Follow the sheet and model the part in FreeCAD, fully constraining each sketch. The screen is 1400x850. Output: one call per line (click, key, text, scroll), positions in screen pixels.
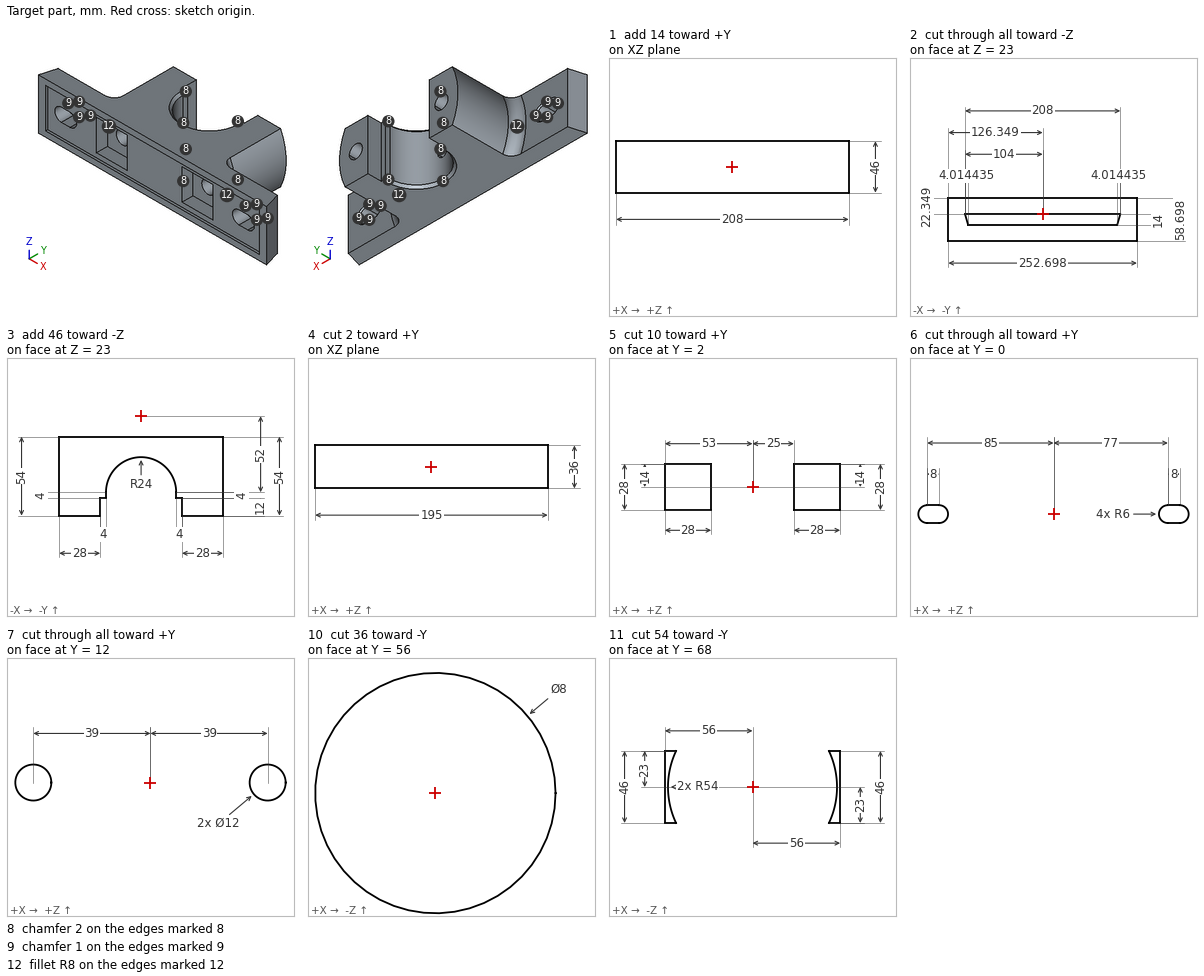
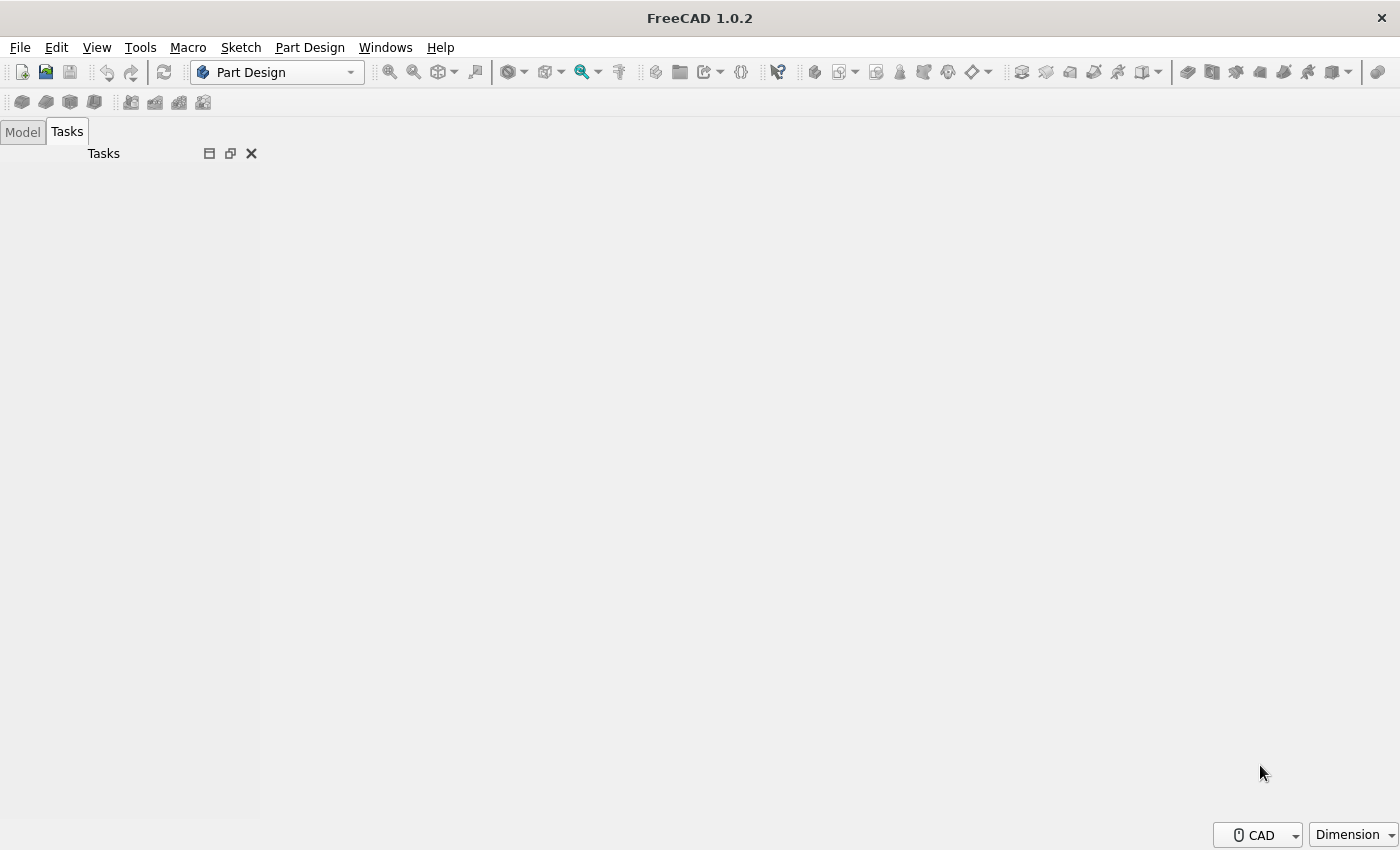
click(22, 72)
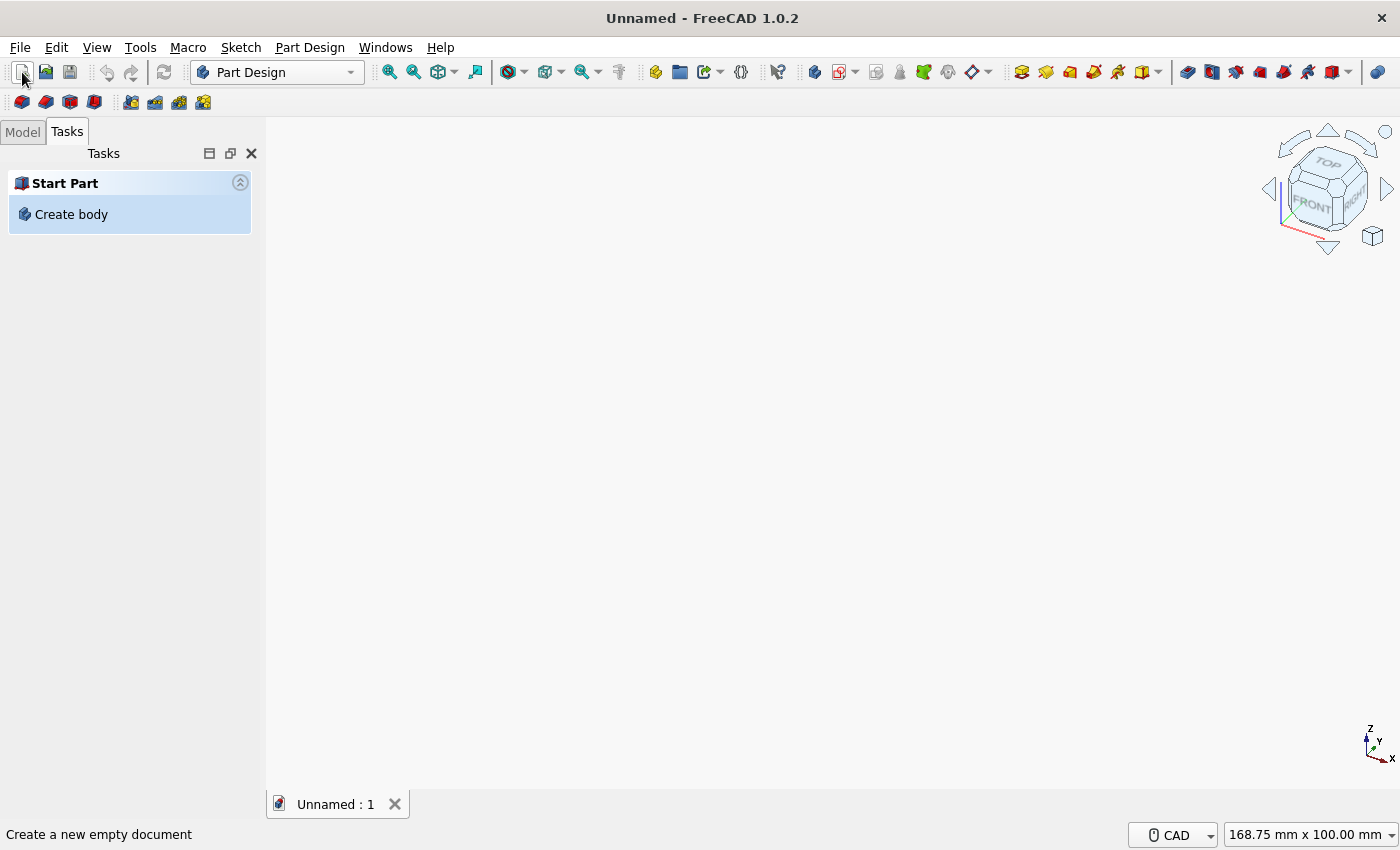
click(840, 72)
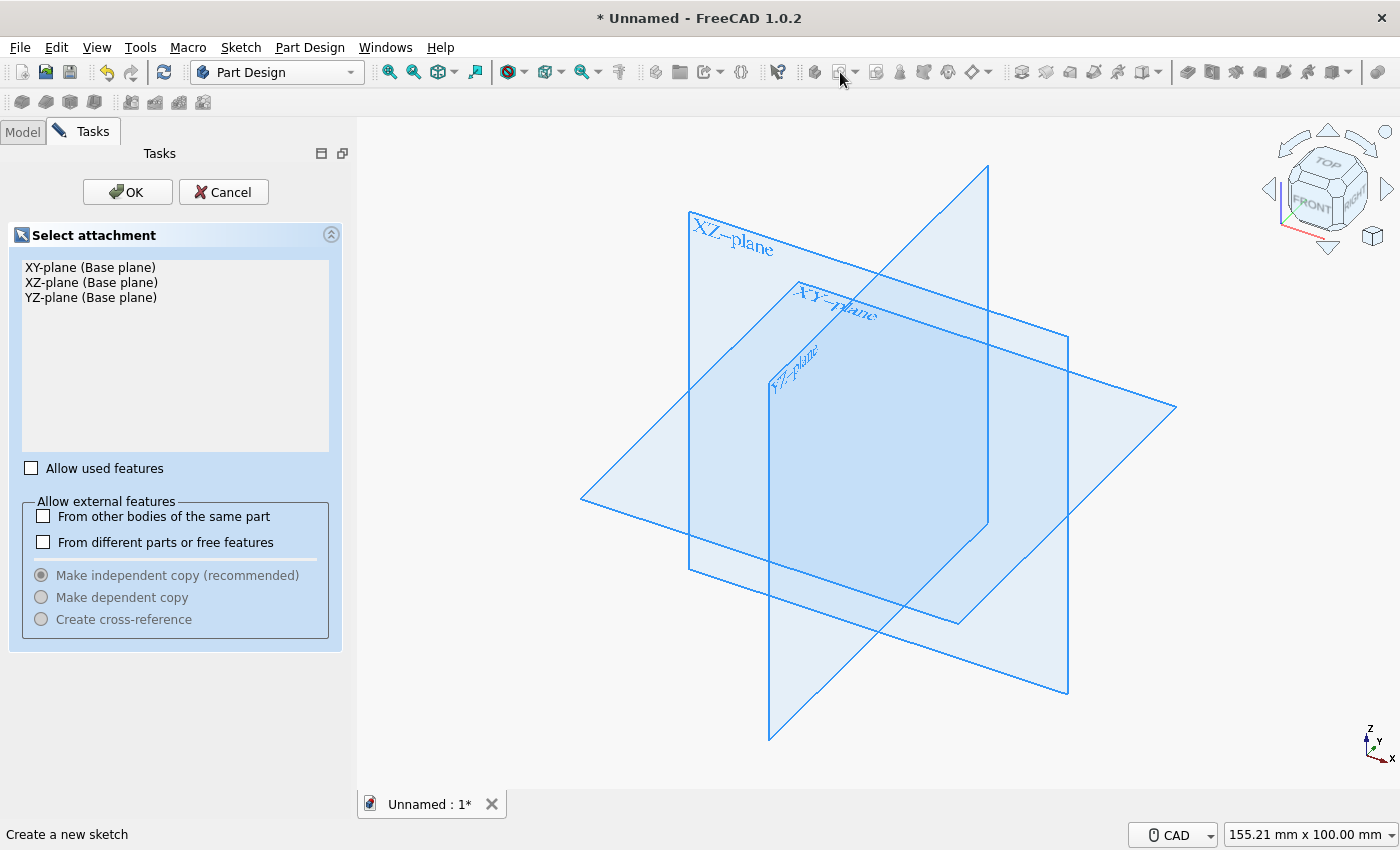
click(82, 282)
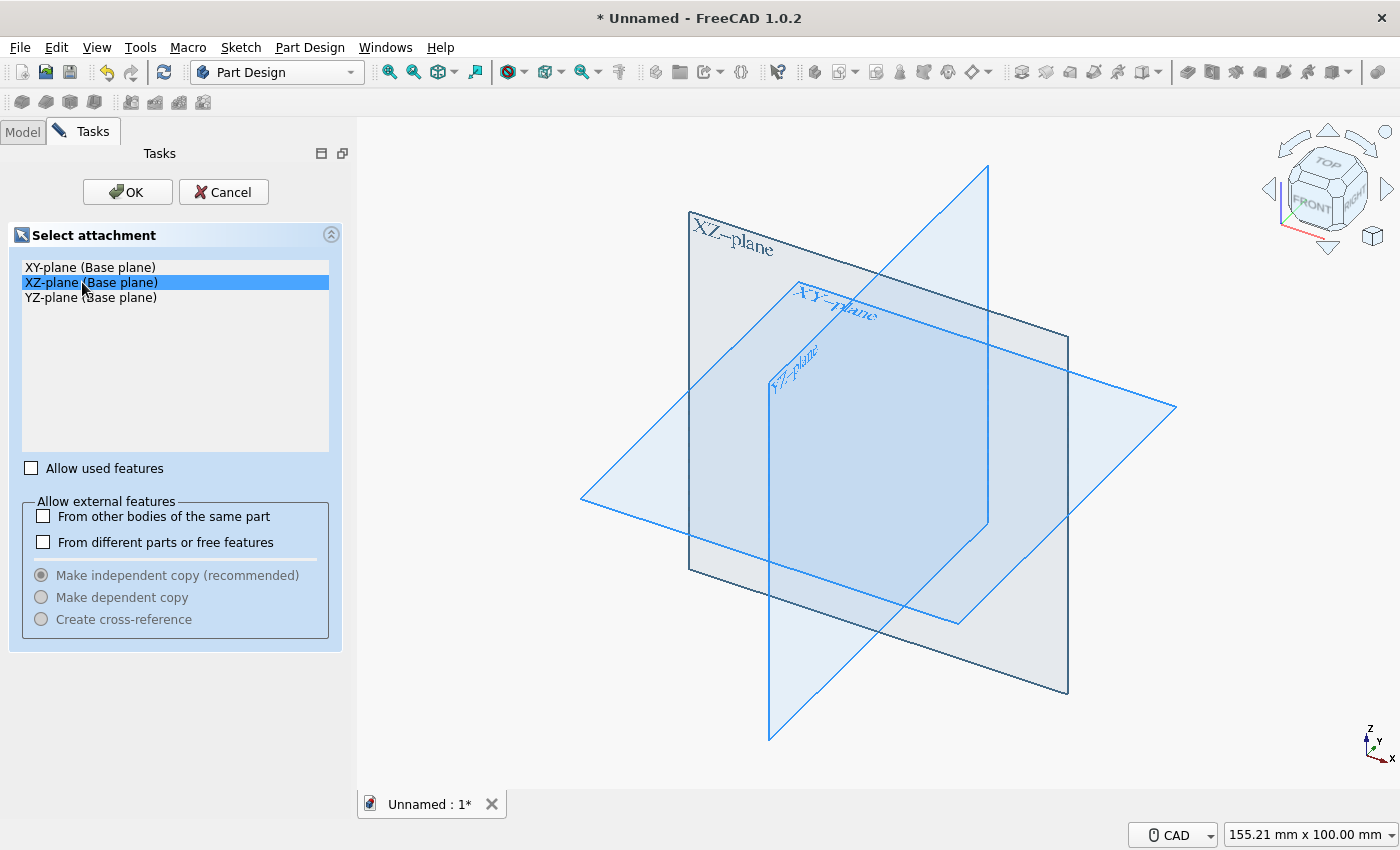
click(128, 192)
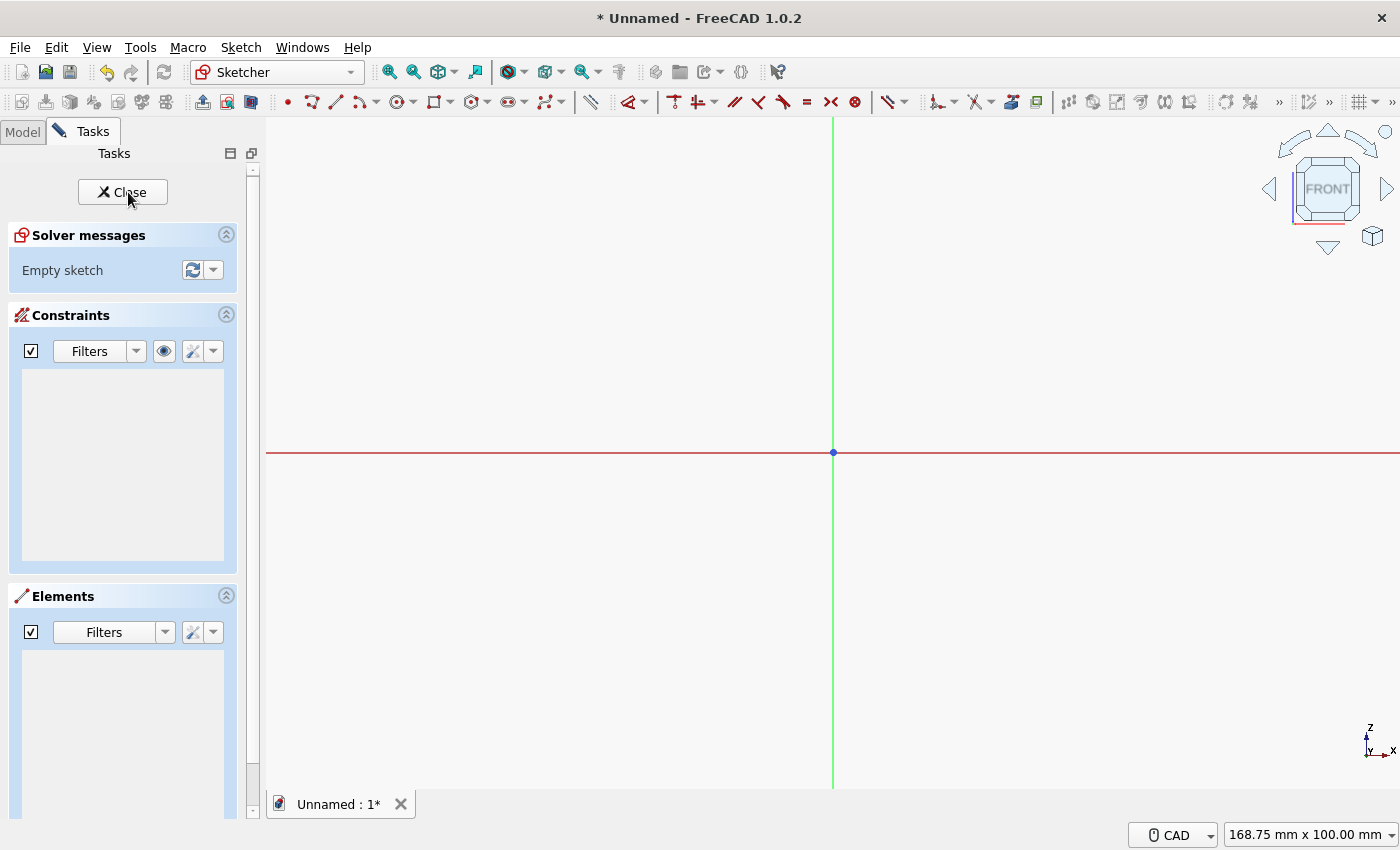
scroll(709, 453, down, 4)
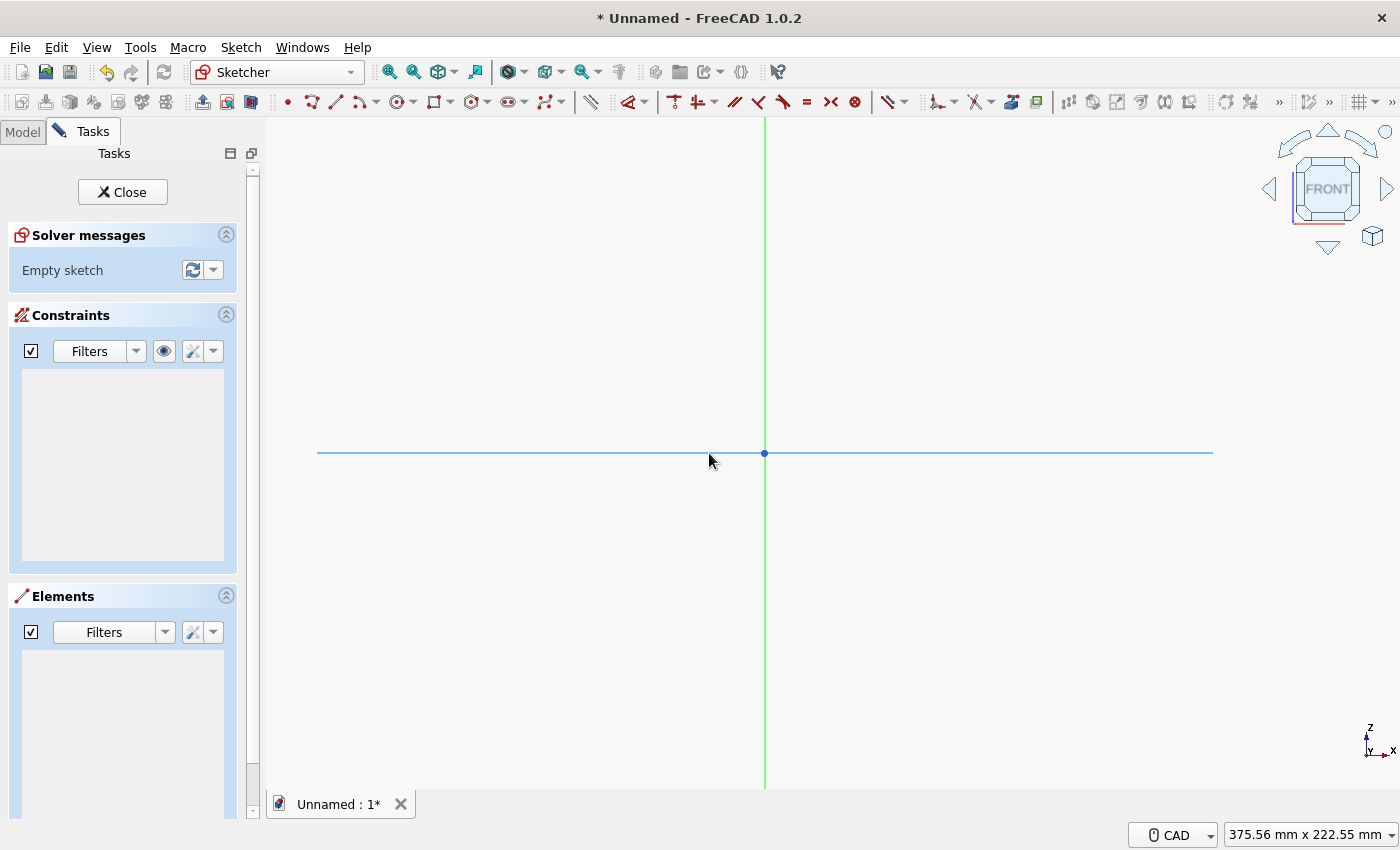
key(g)
key(v)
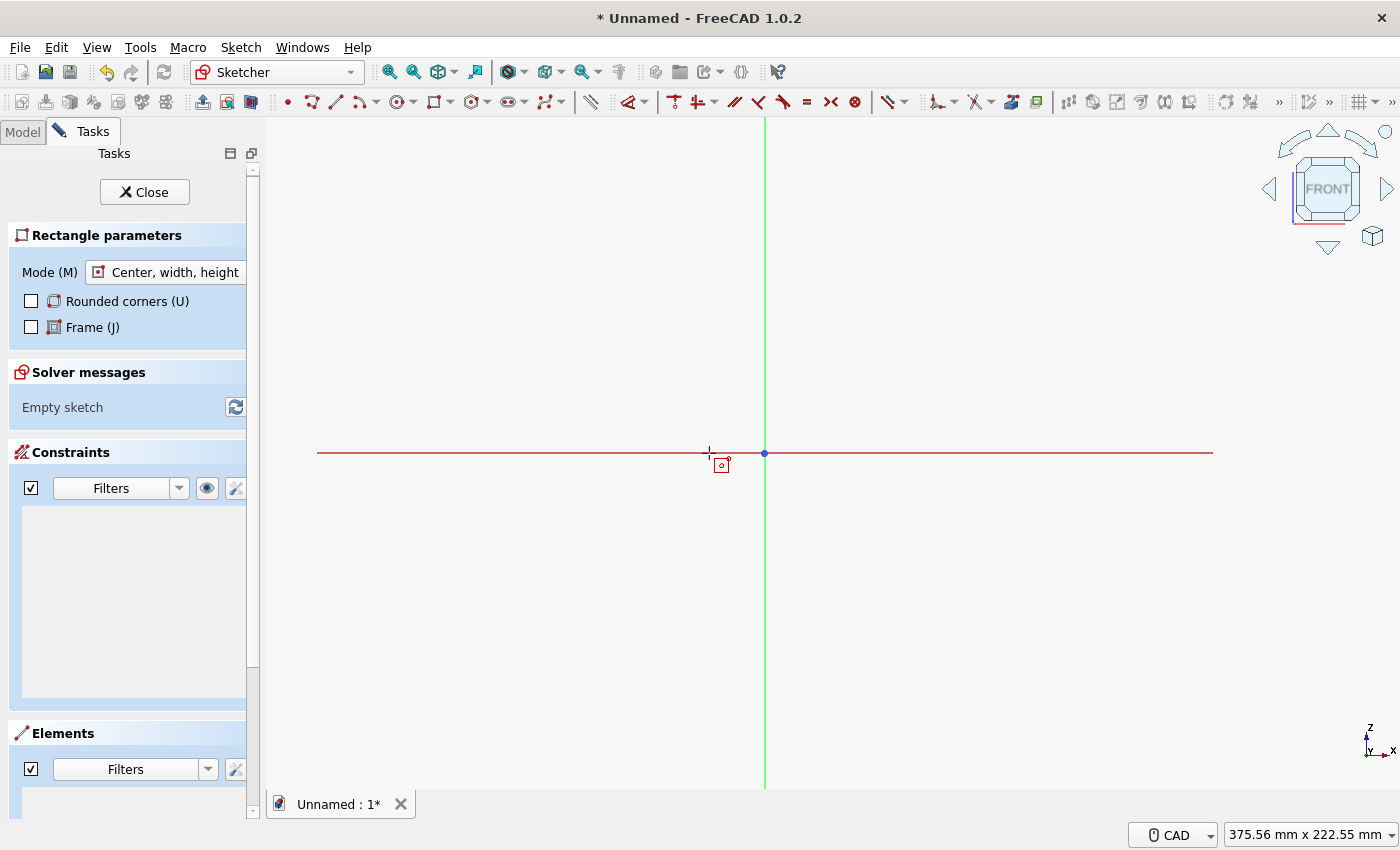
click(765, 453)
move(1079, 384)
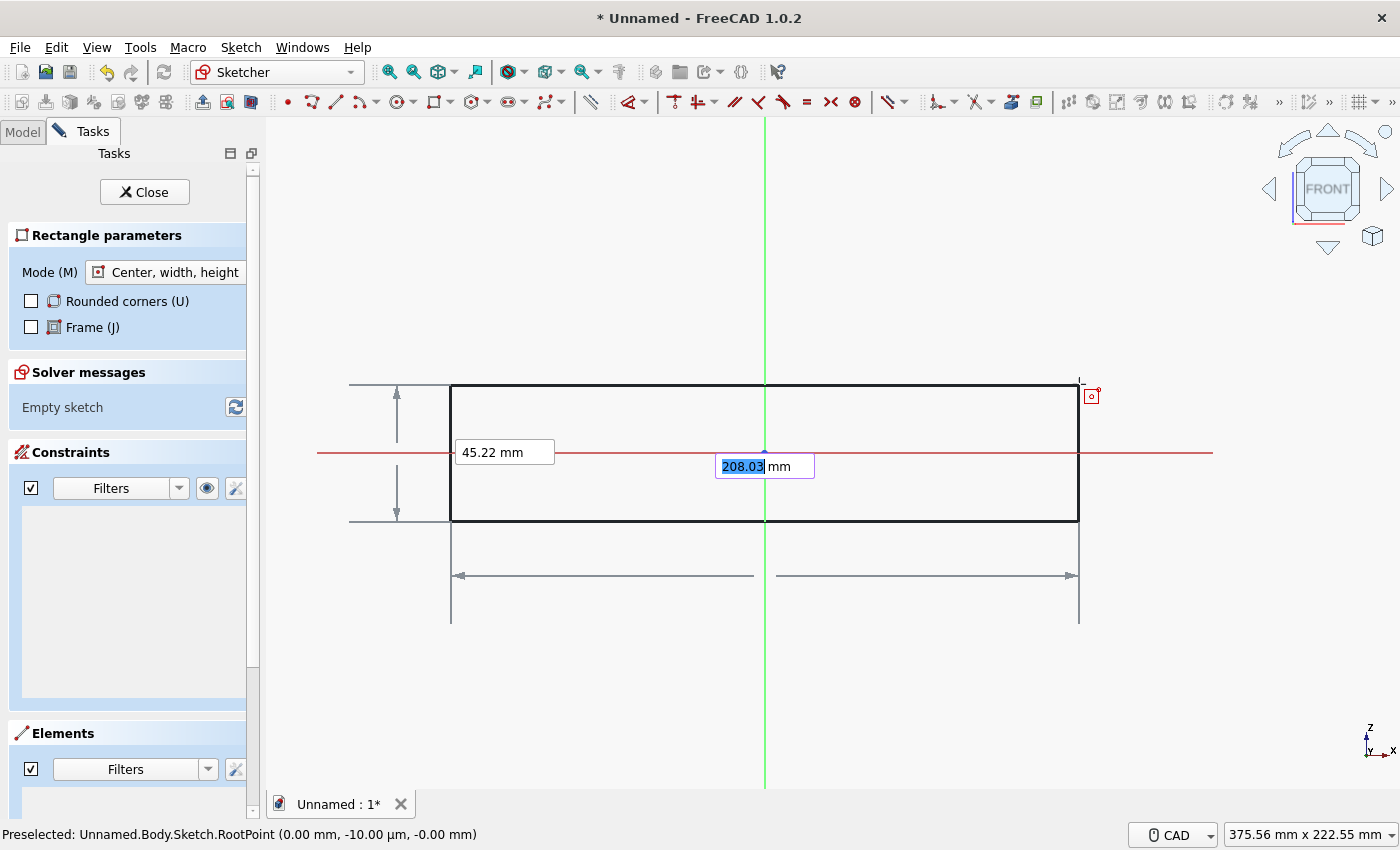
text(208)
key(Tab)
text(46)
key(Return)
key(Escape)